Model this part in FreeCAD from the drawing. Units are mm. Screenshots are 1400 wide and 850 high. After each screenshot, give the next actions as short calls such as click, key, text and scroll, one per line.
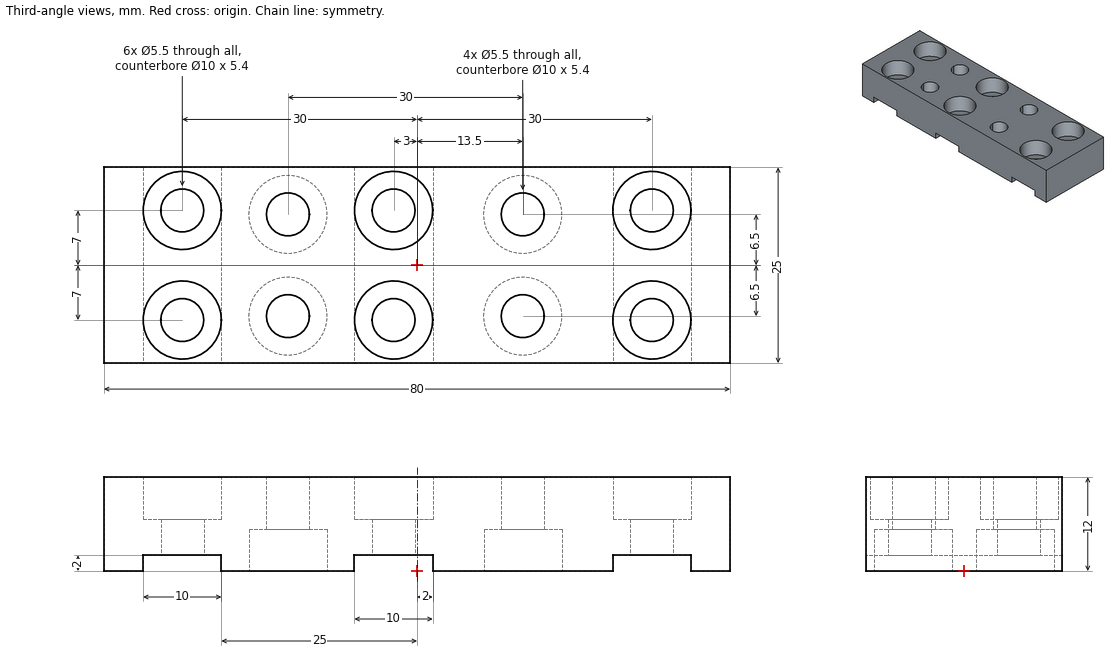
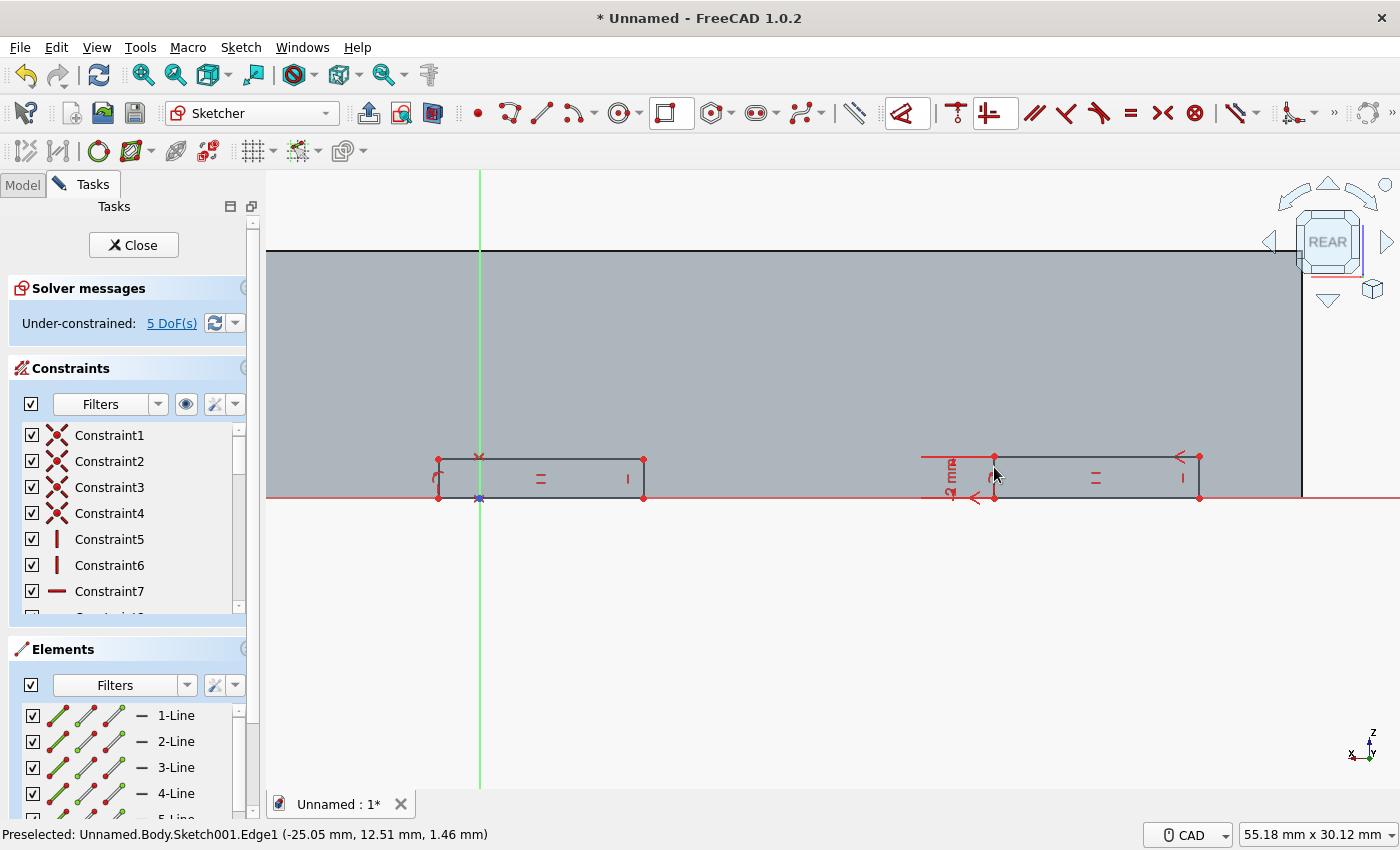
click(439, 467)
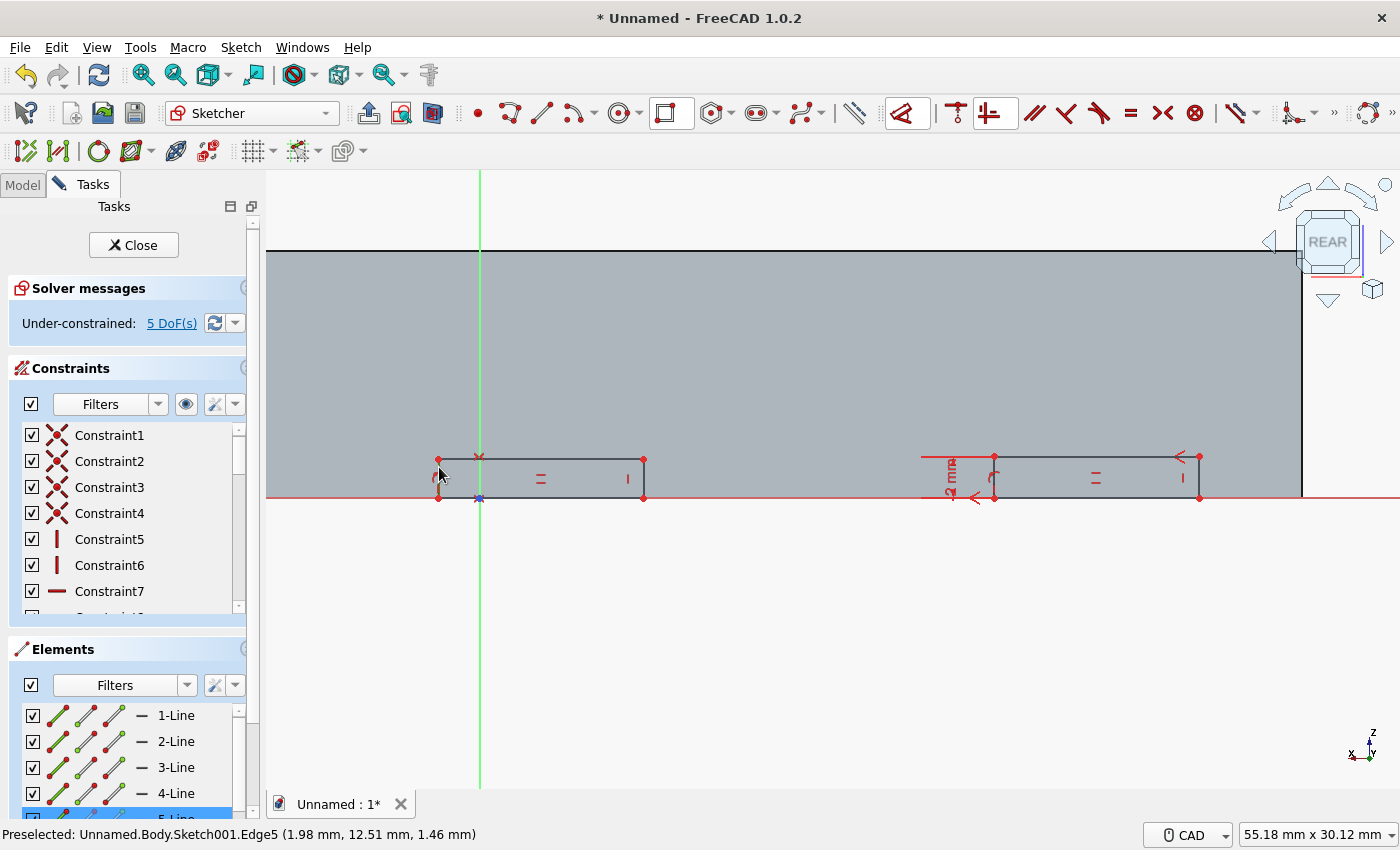
key(i)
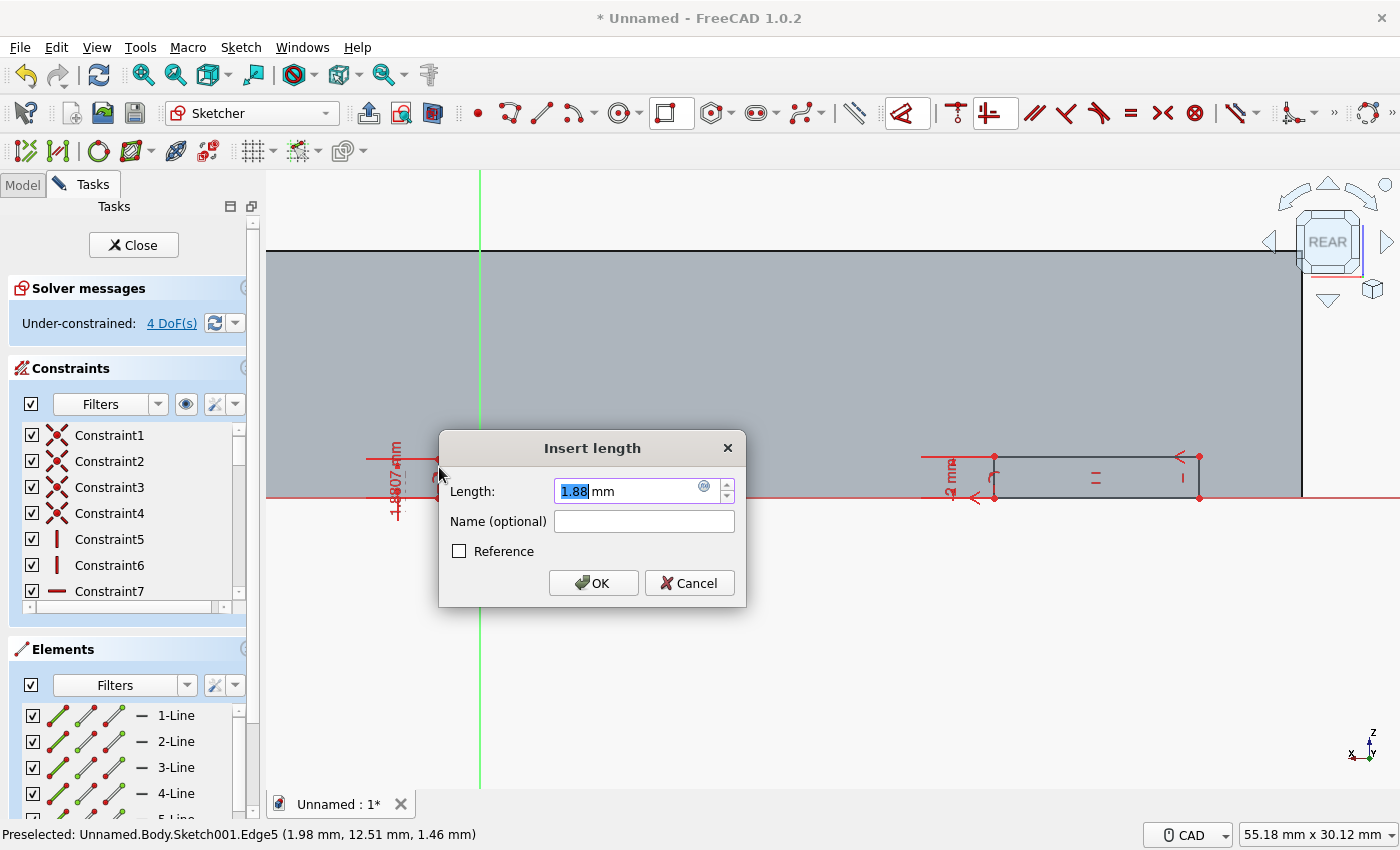
text(2)
key(Return)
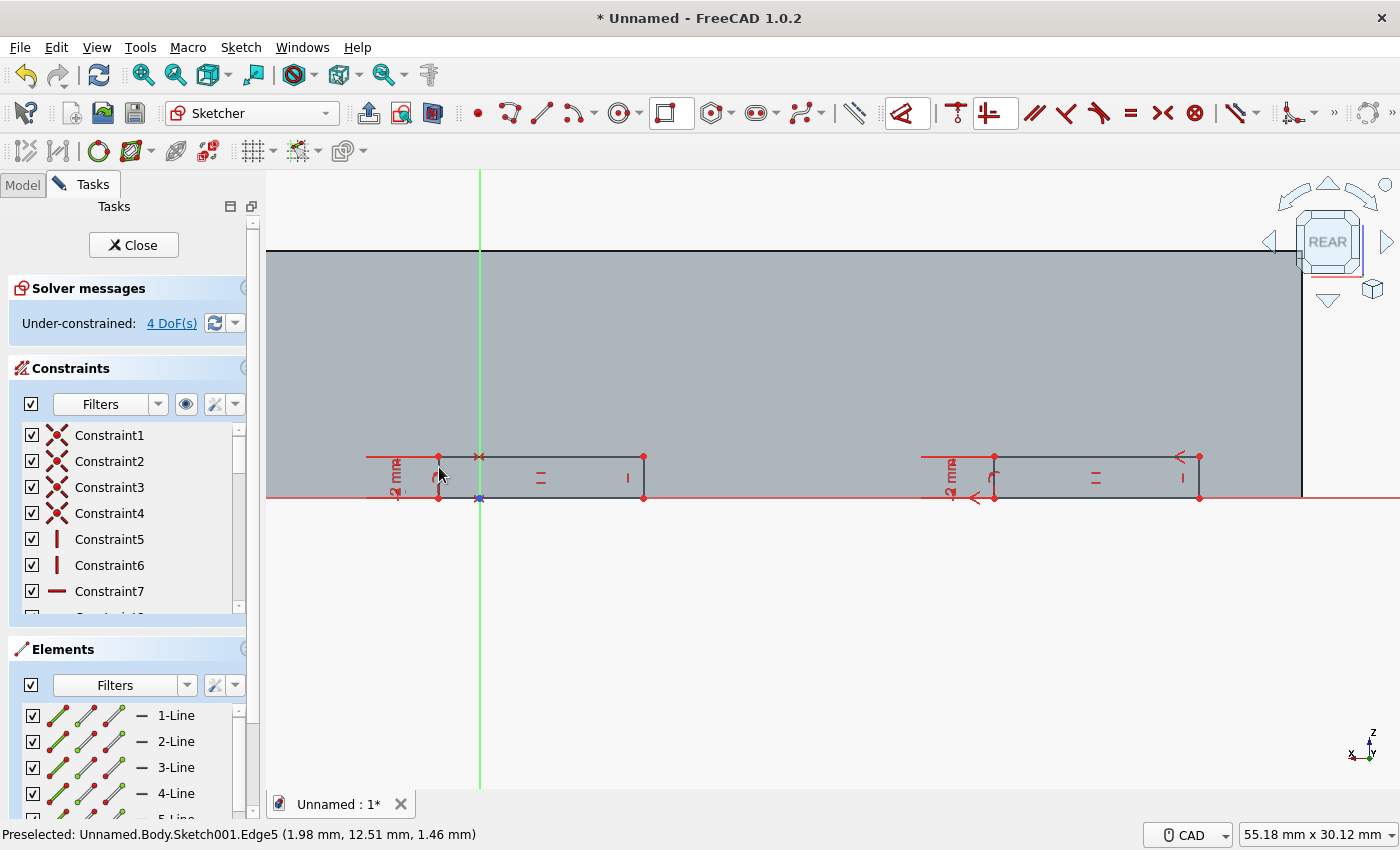
click(1056, 498)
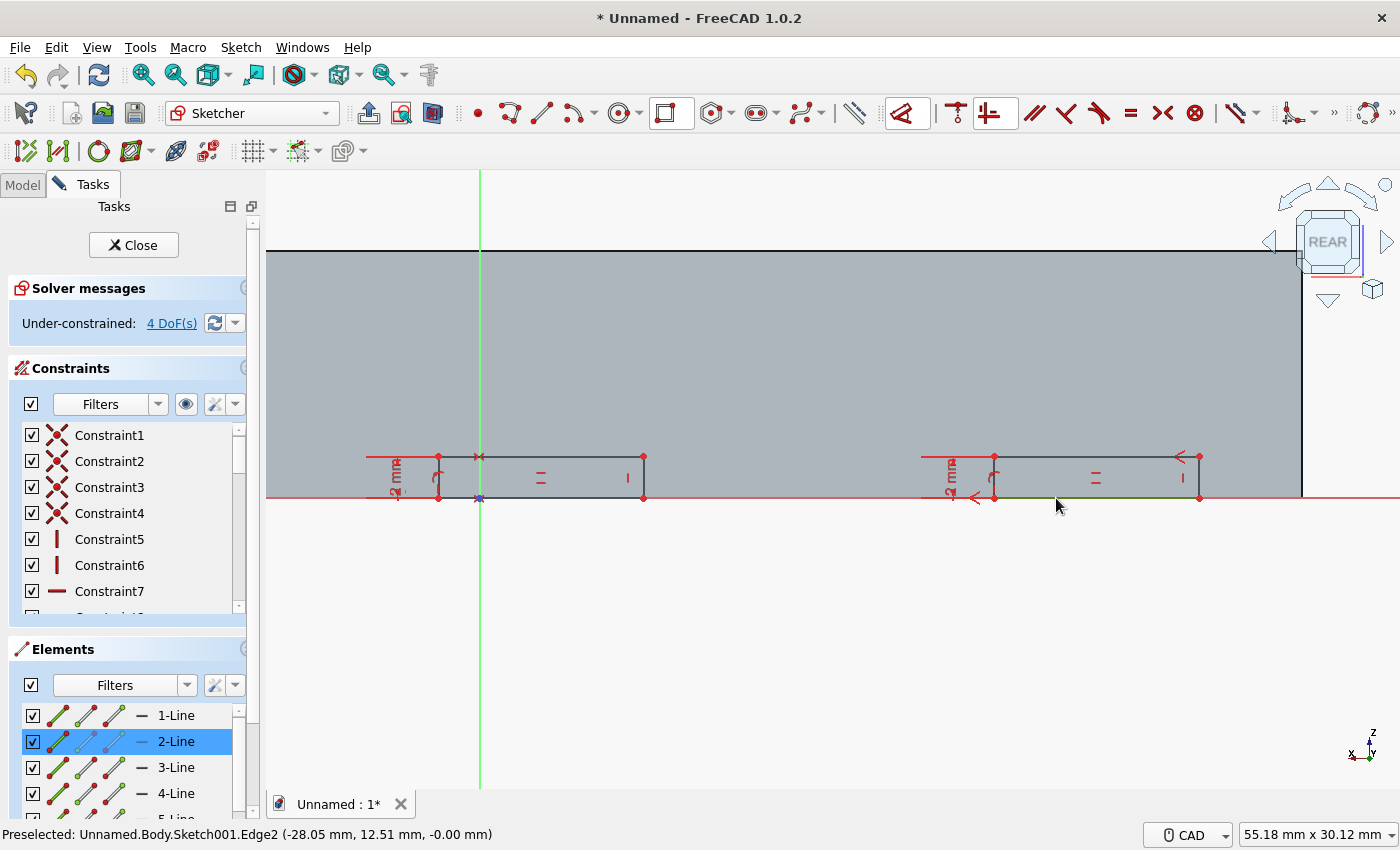
click(924, 114)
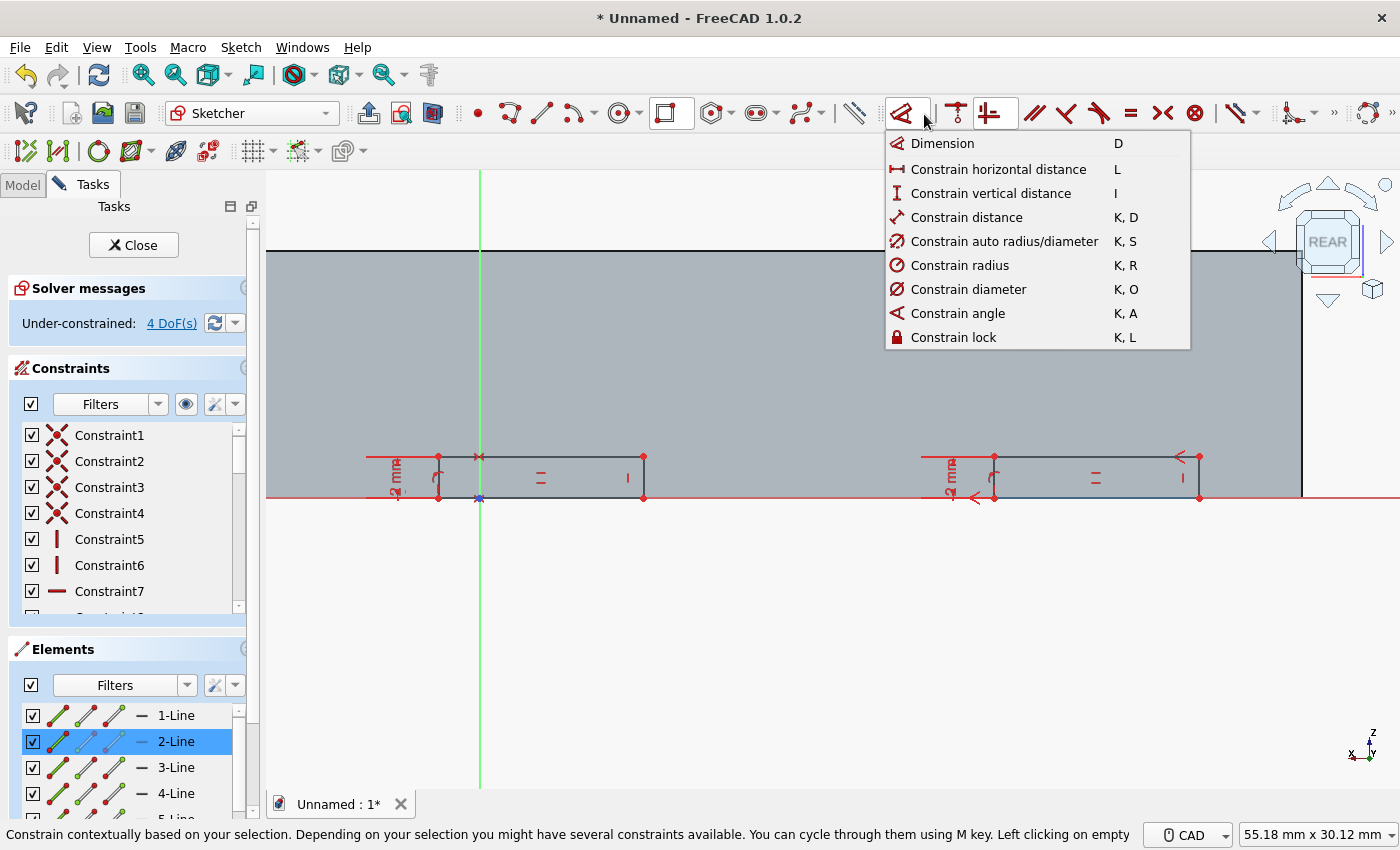
click(1038, 169)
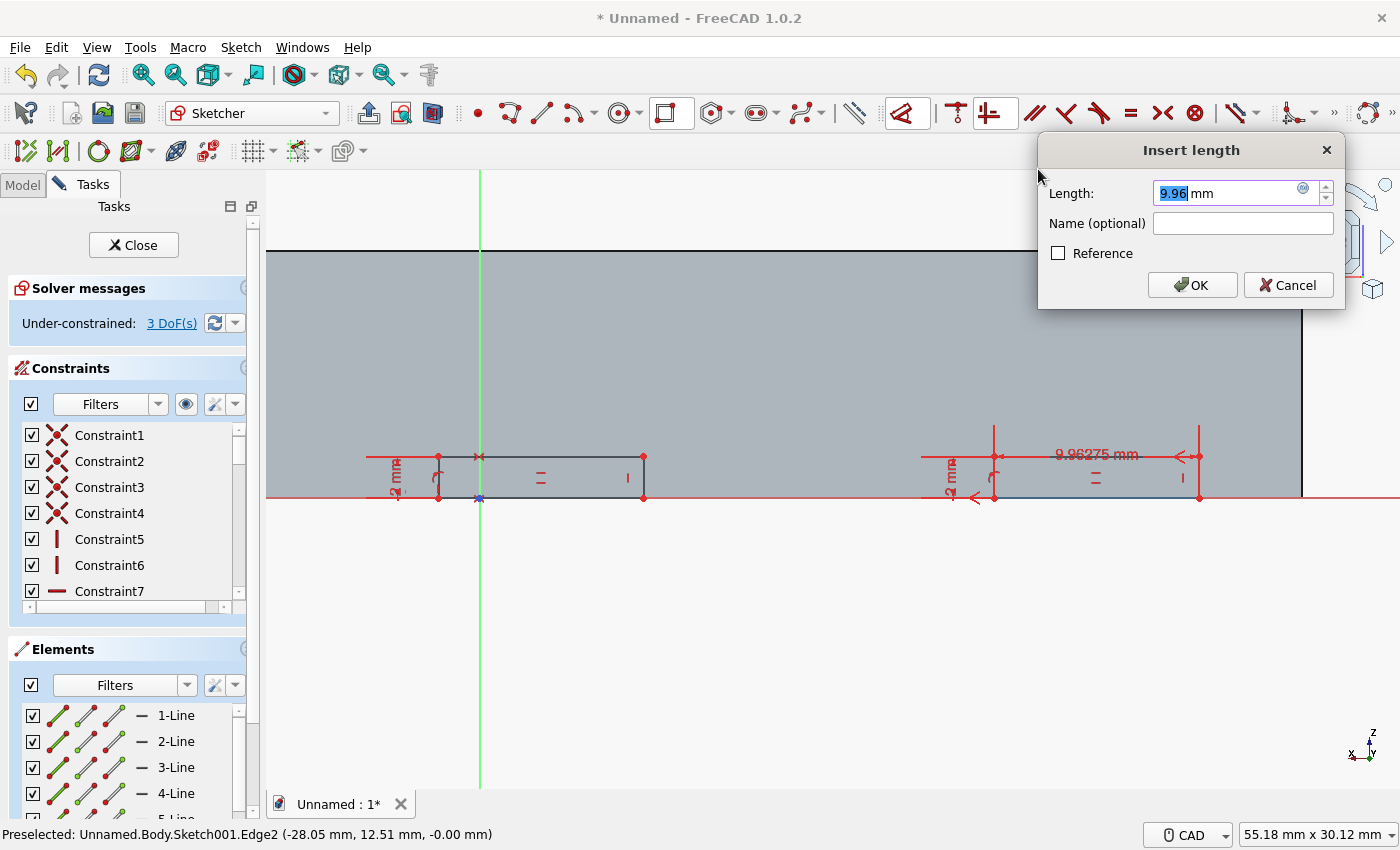
text(10)
key(Return)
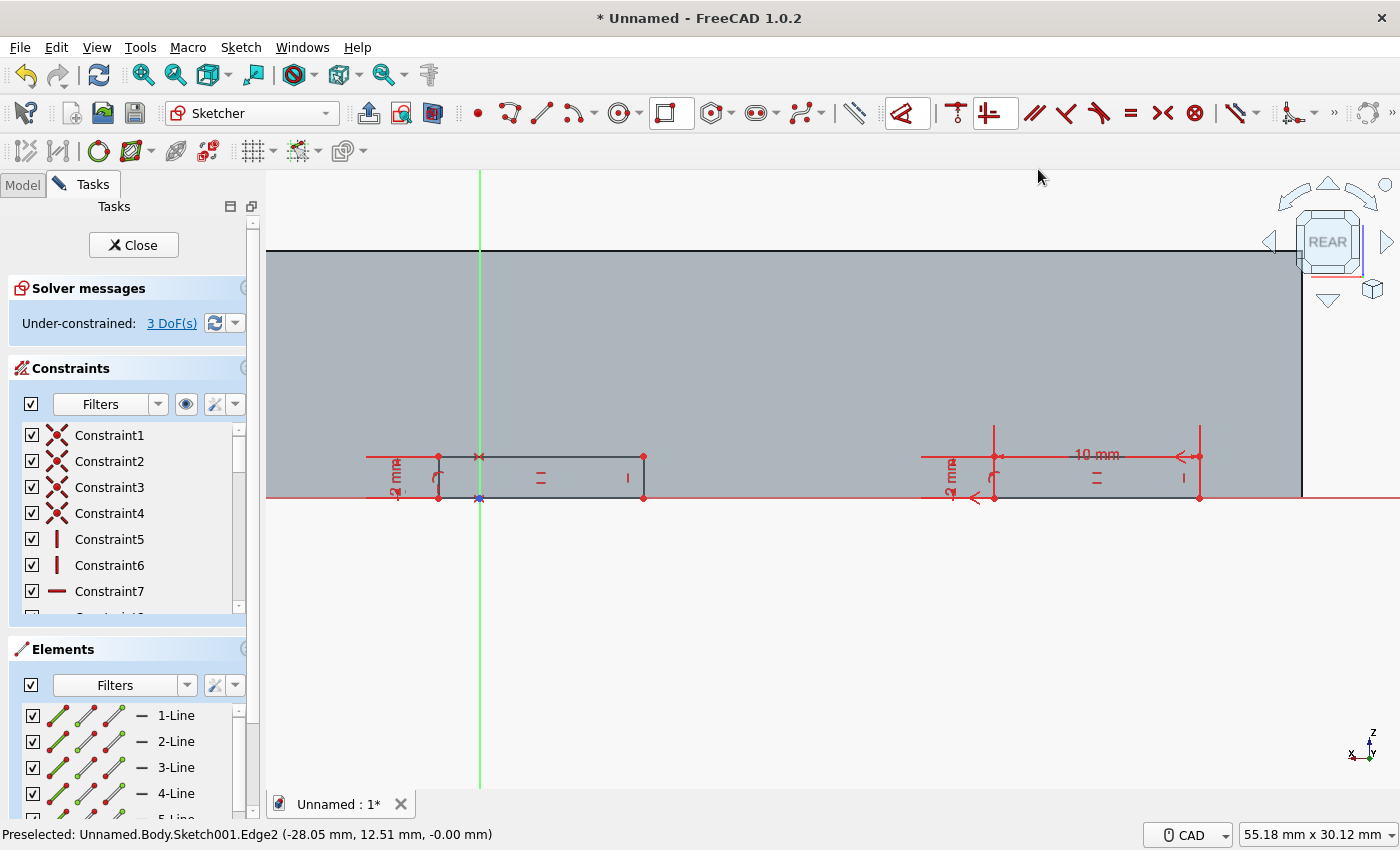
click(500, 498)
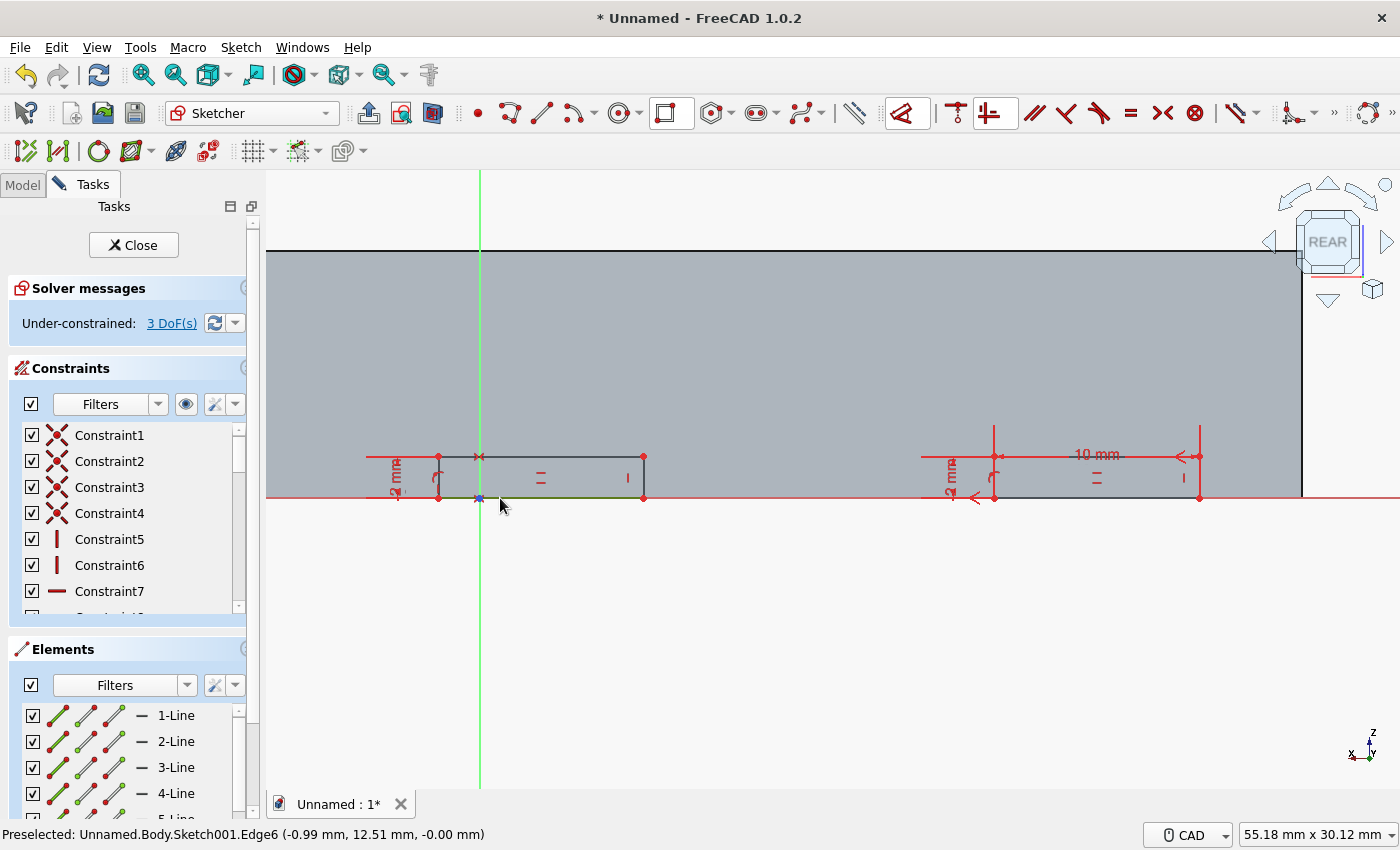
key(l)